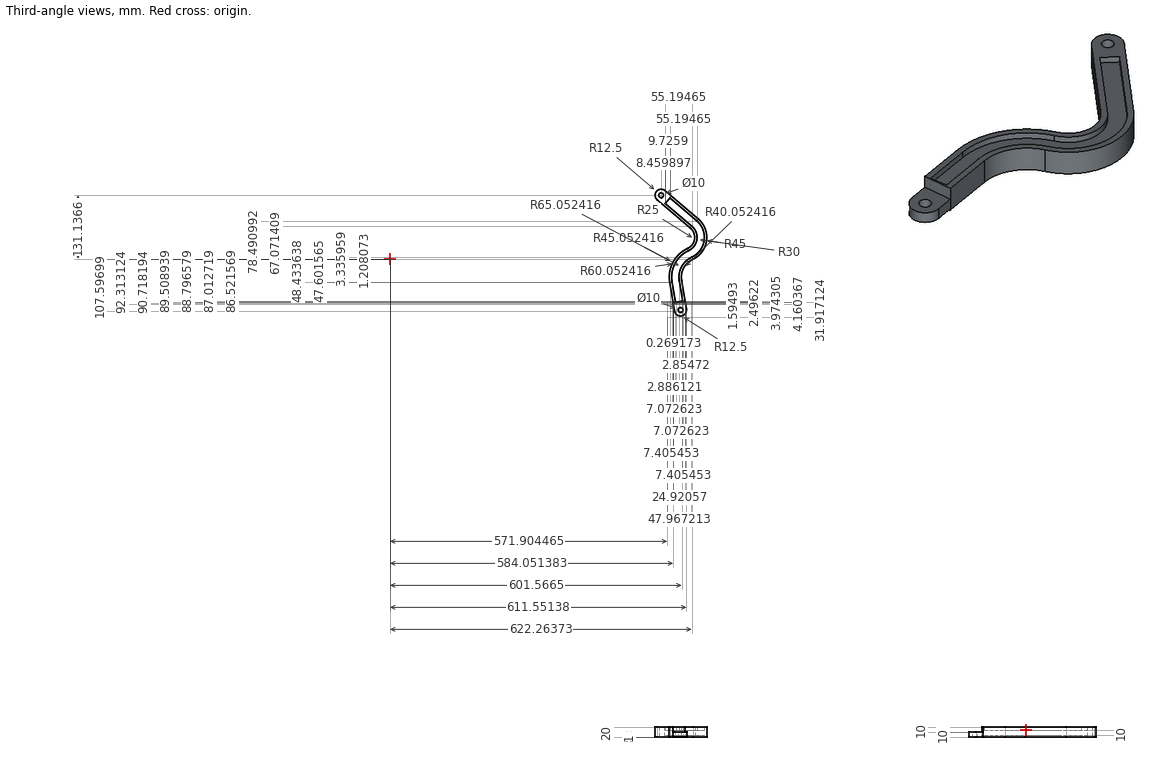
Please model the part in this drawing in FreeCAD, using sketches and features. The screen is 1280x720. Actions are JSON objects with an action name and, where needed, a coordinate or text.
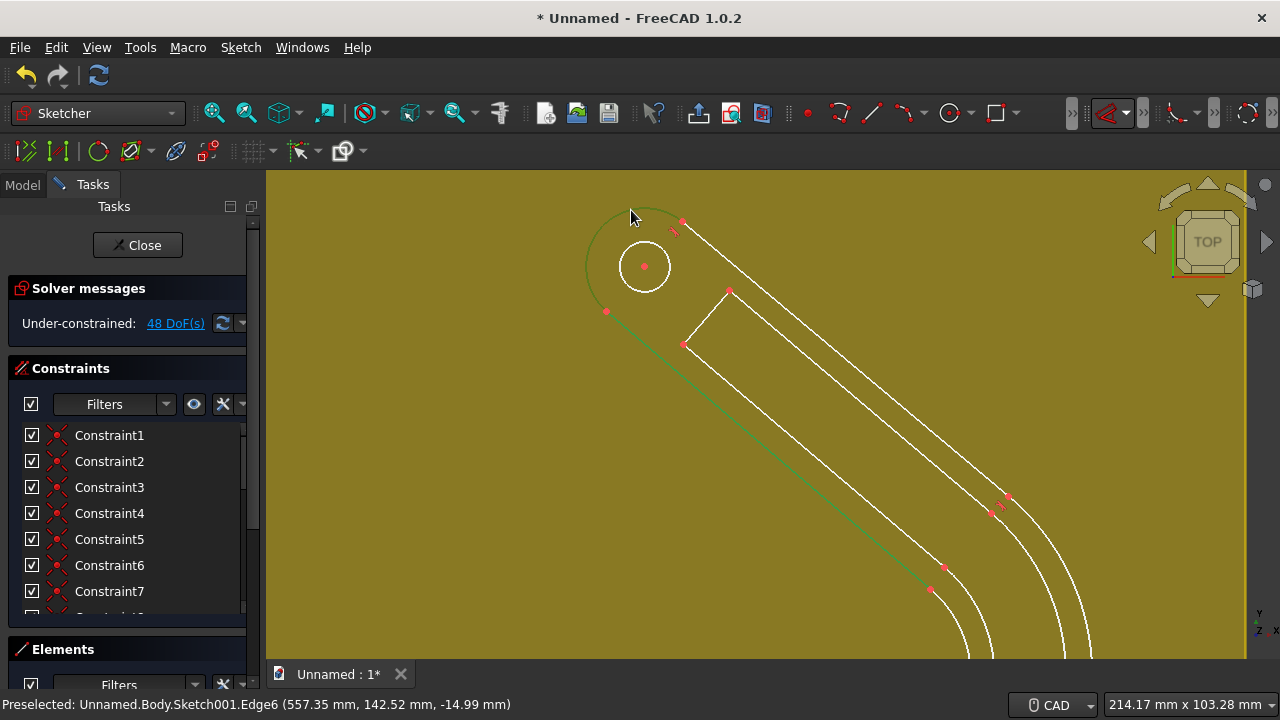
{"action": "key", "text": "t"}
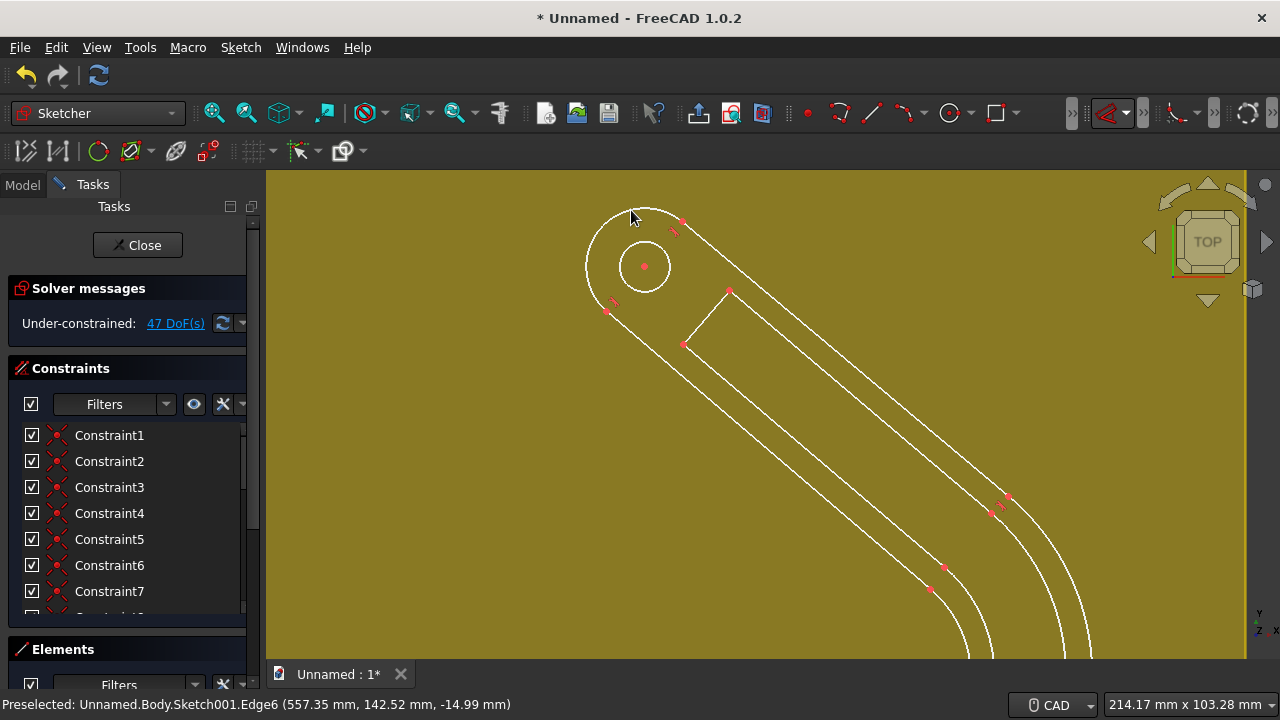
{"action": "left_click", "coordinate": [704, 395]}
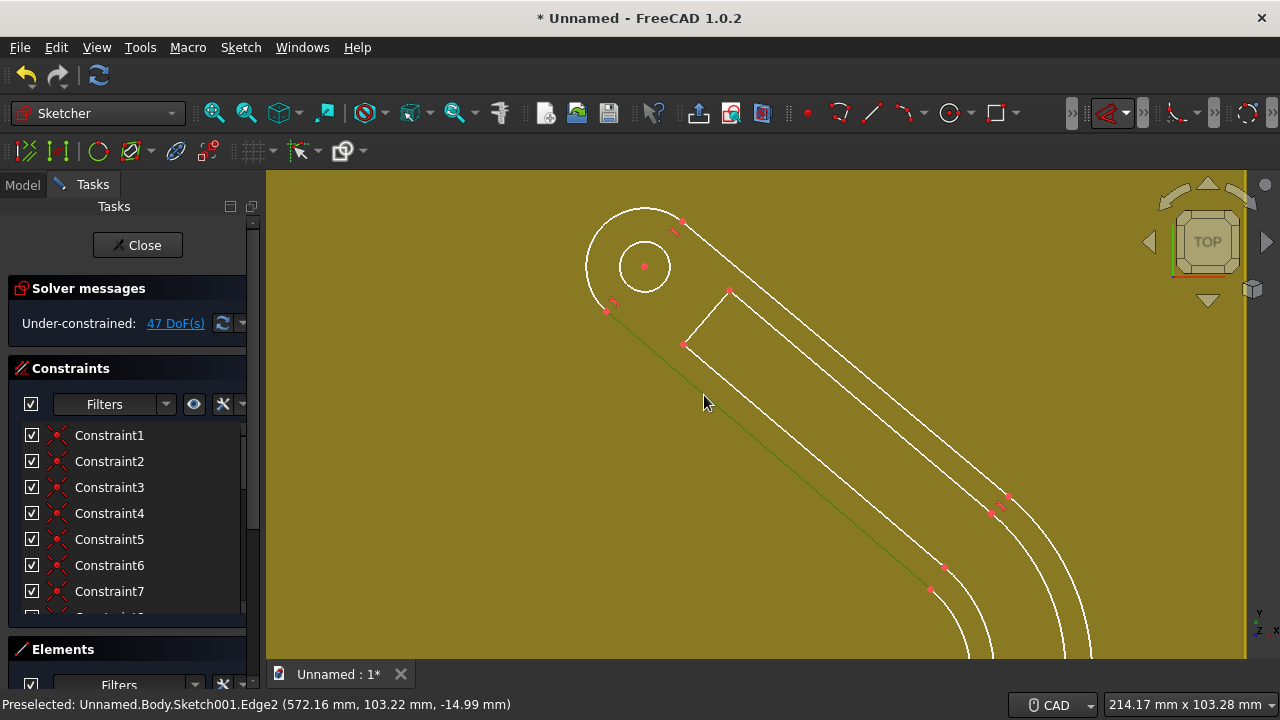
{"action": "left_click", "coordinate": [959, 626]}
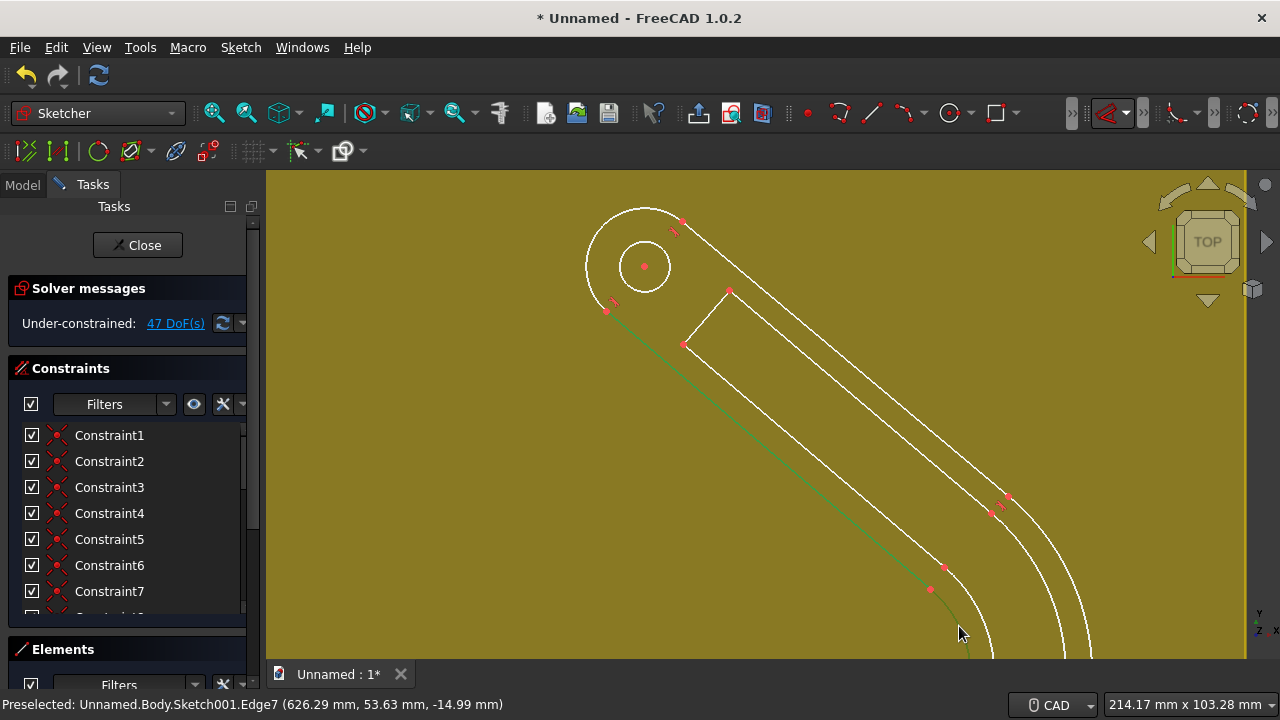
{"action": "key", "text": "t"}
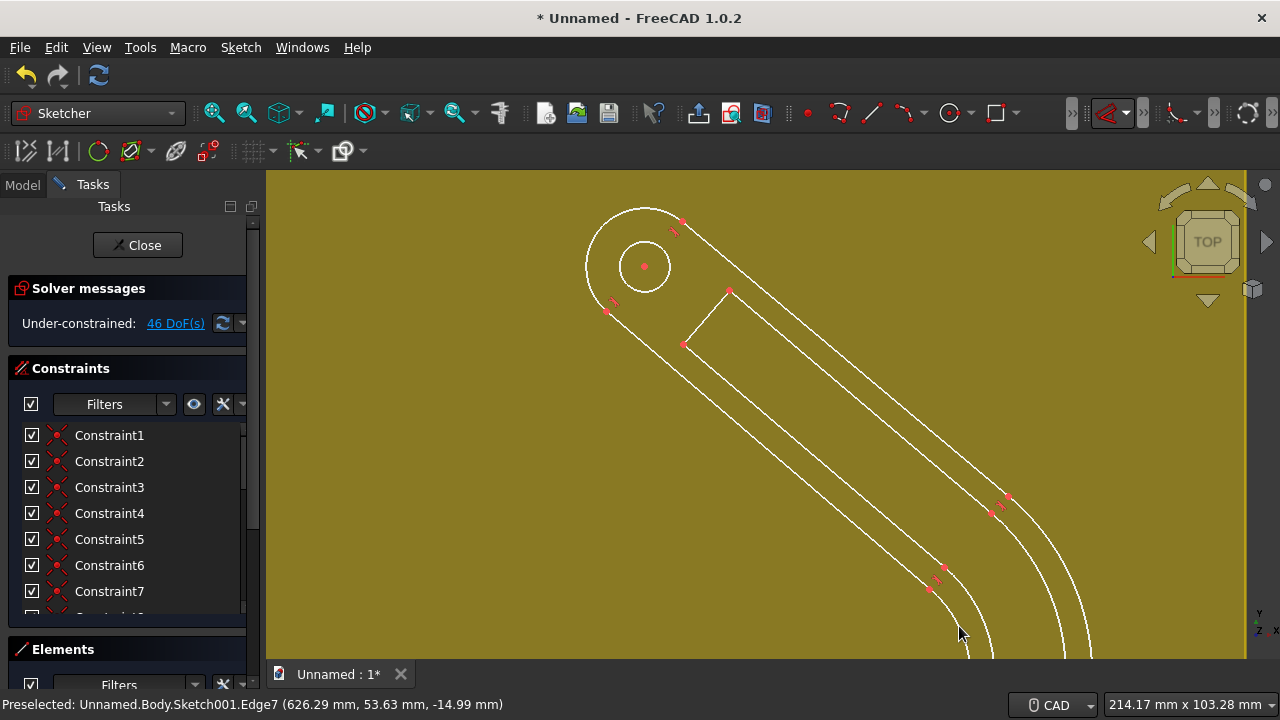
{"action": "scroll", "coordinate": [645, 261], "scroll_direction": "down", "scroll_amount": 6}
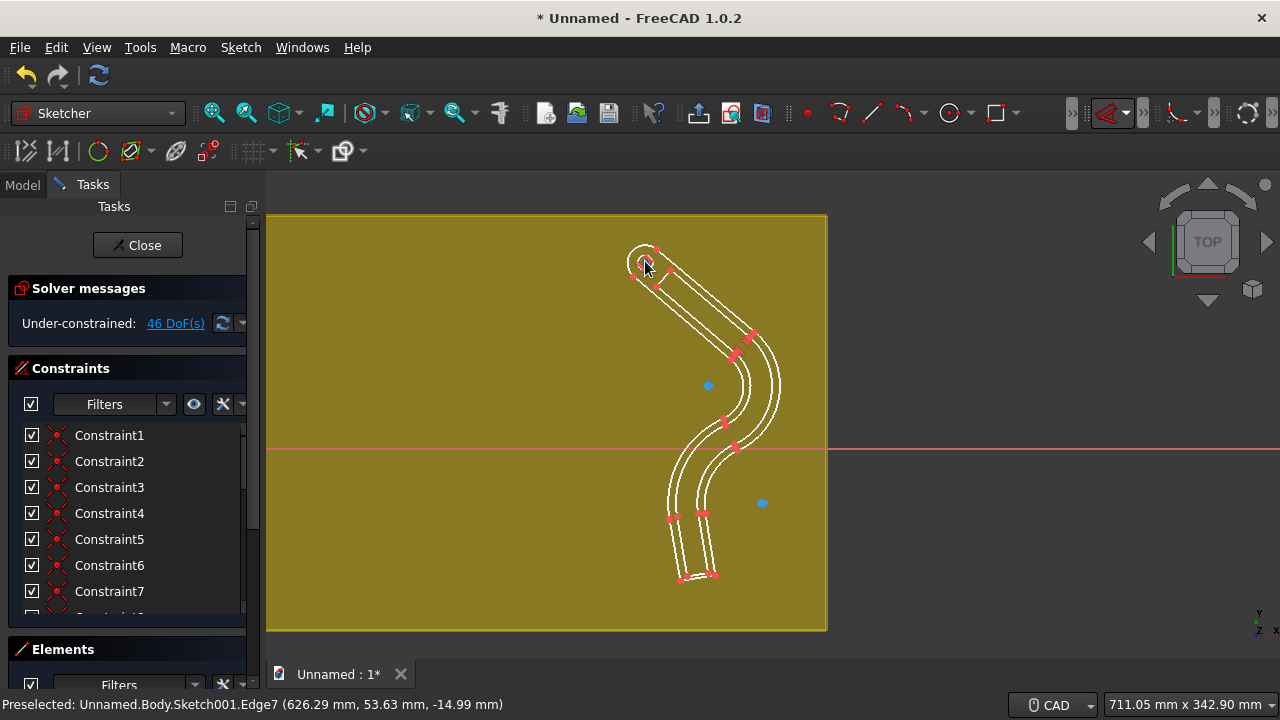
{"action": "scroll", "coordinate": [673, 538], "scroll_direction": "up", "scroll_amount": 3}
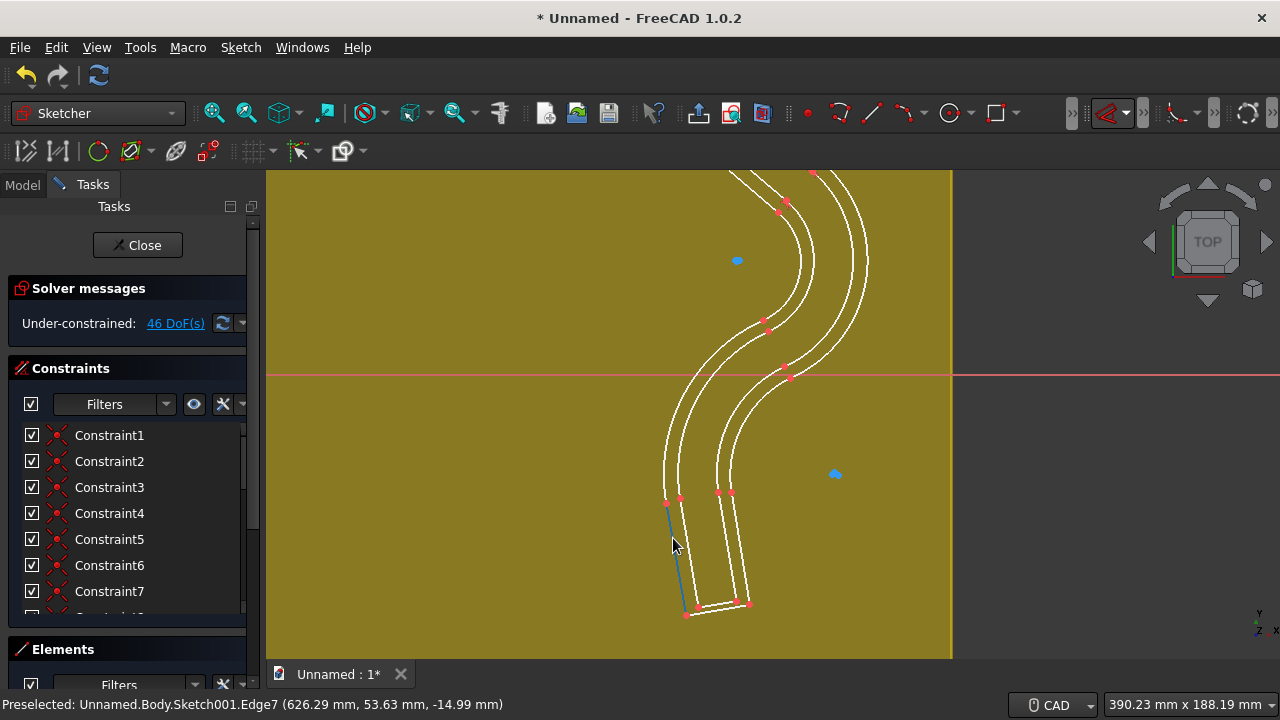
{"action": "left_click", "coordinate": [672, 537]}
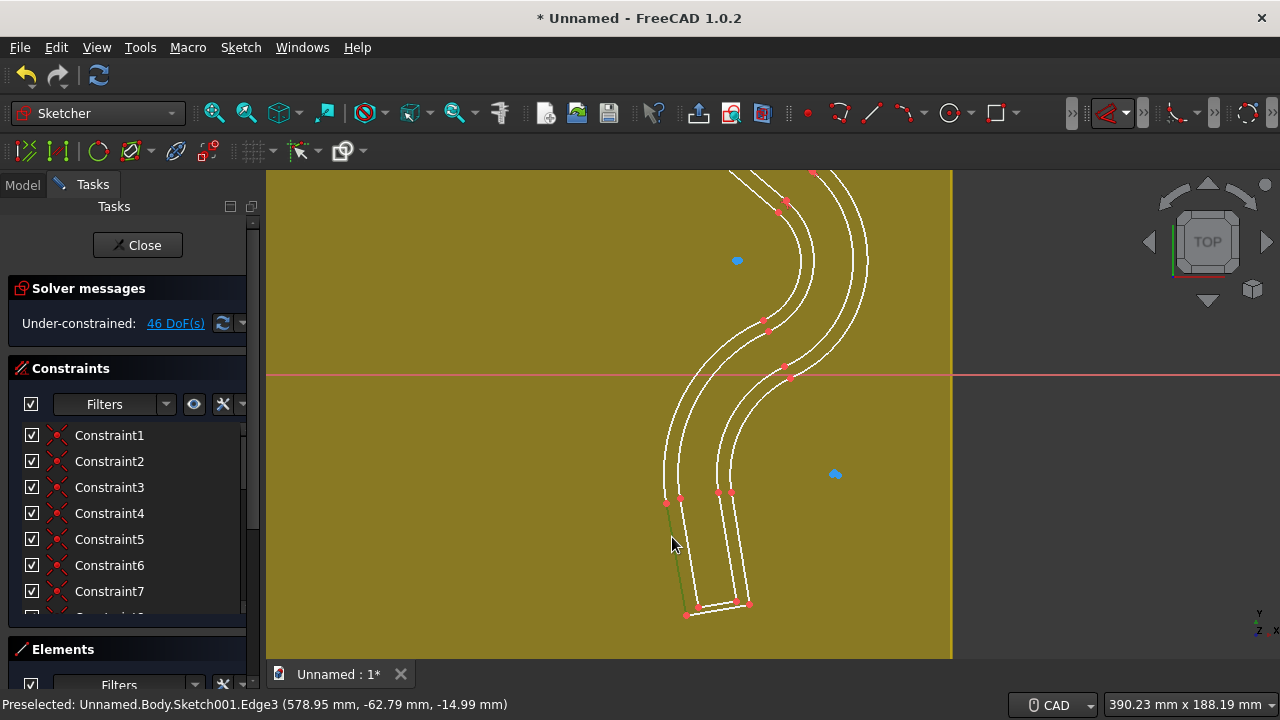
{"action": "left_click", "coordinate": [710, 359]}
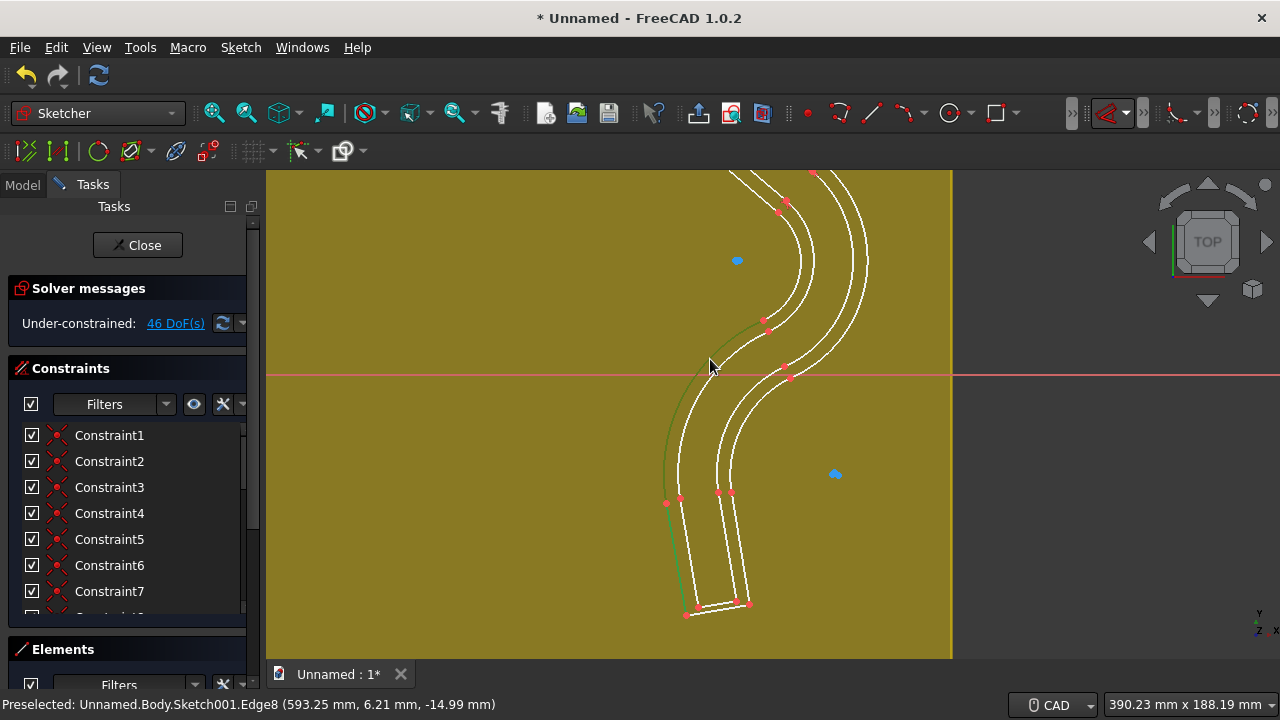
{"action": "key", "text": "t"}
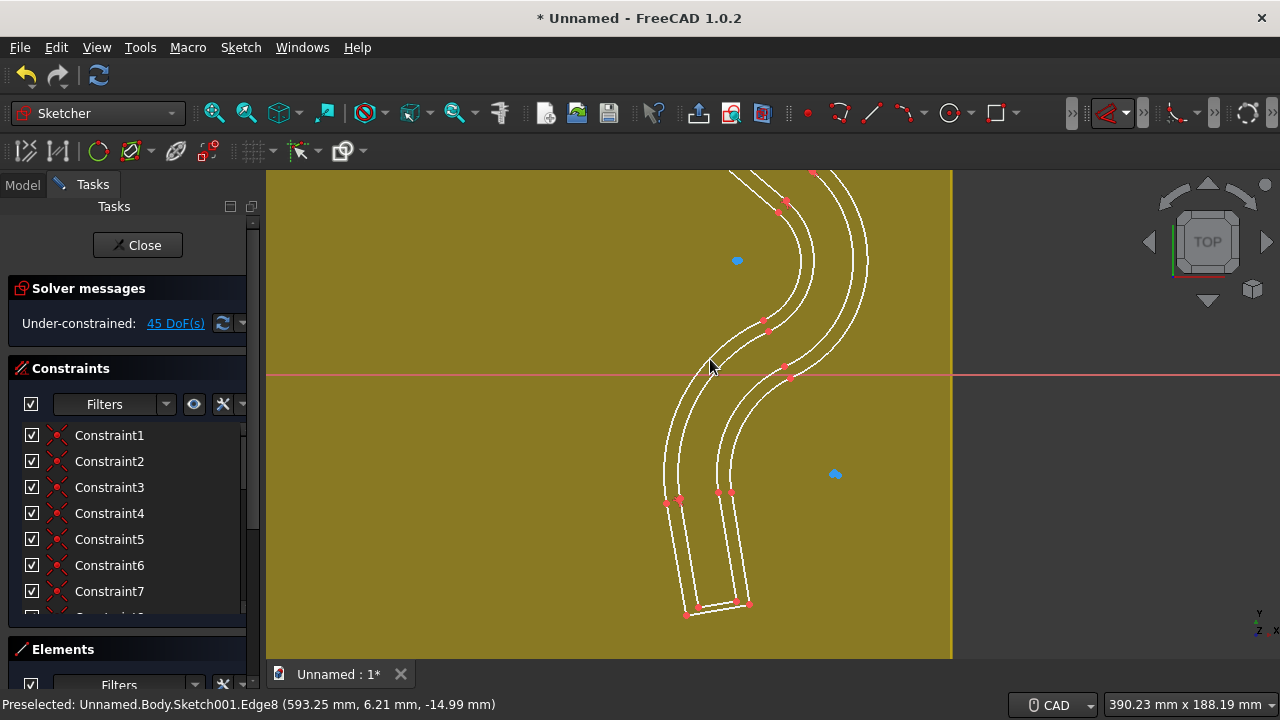
{"action": "left_click", "coordinate": [744, 571]}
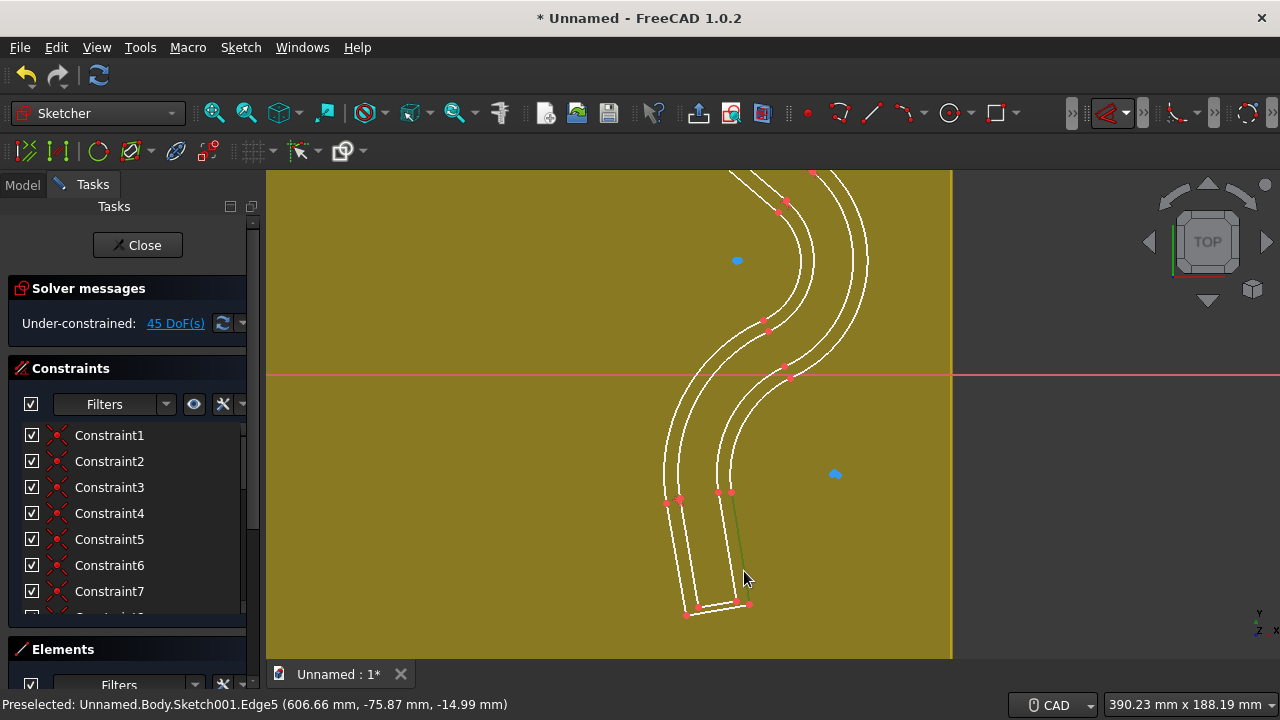
{"action": "left_click", "coordinate": [758, 403]}